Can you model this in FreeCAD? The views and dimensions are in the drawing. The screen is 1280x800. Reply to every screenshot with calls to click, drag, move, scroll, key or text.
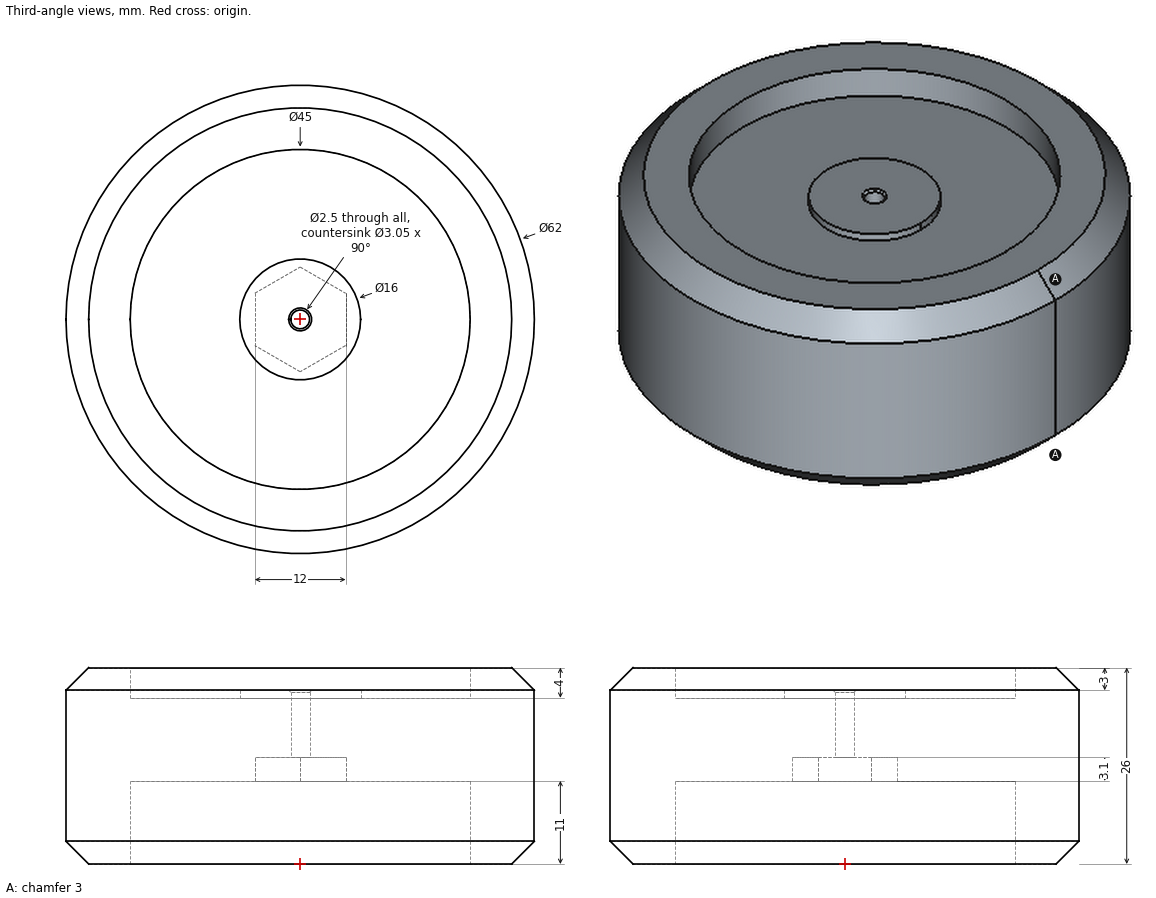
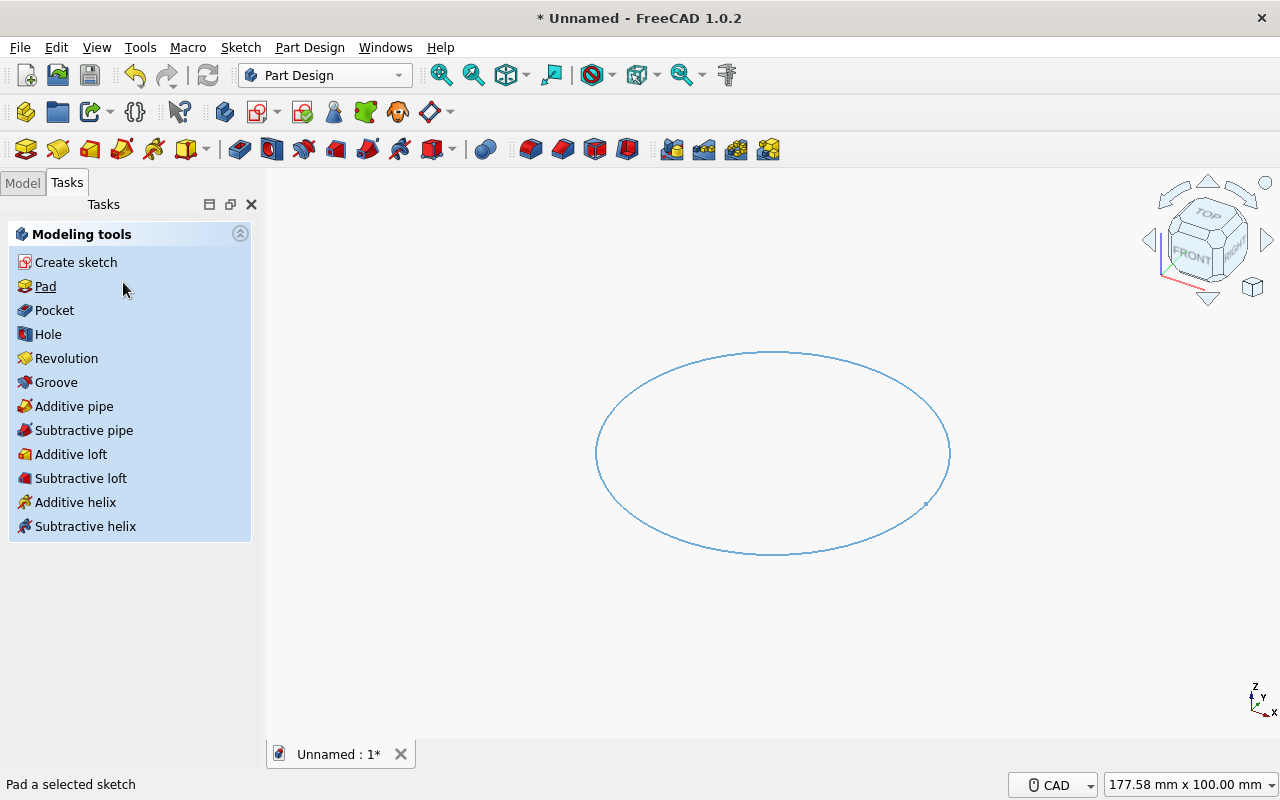
click(26, 150)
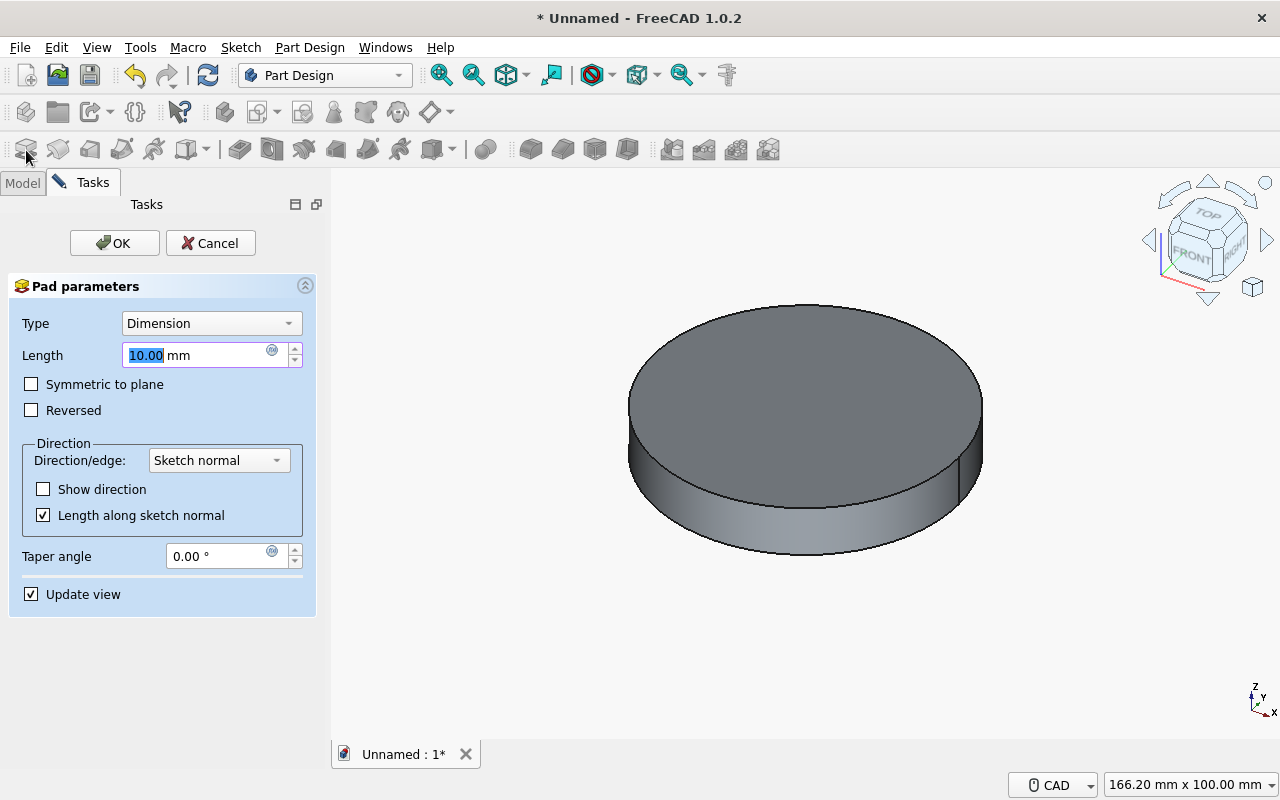
text(26)
key(Tab)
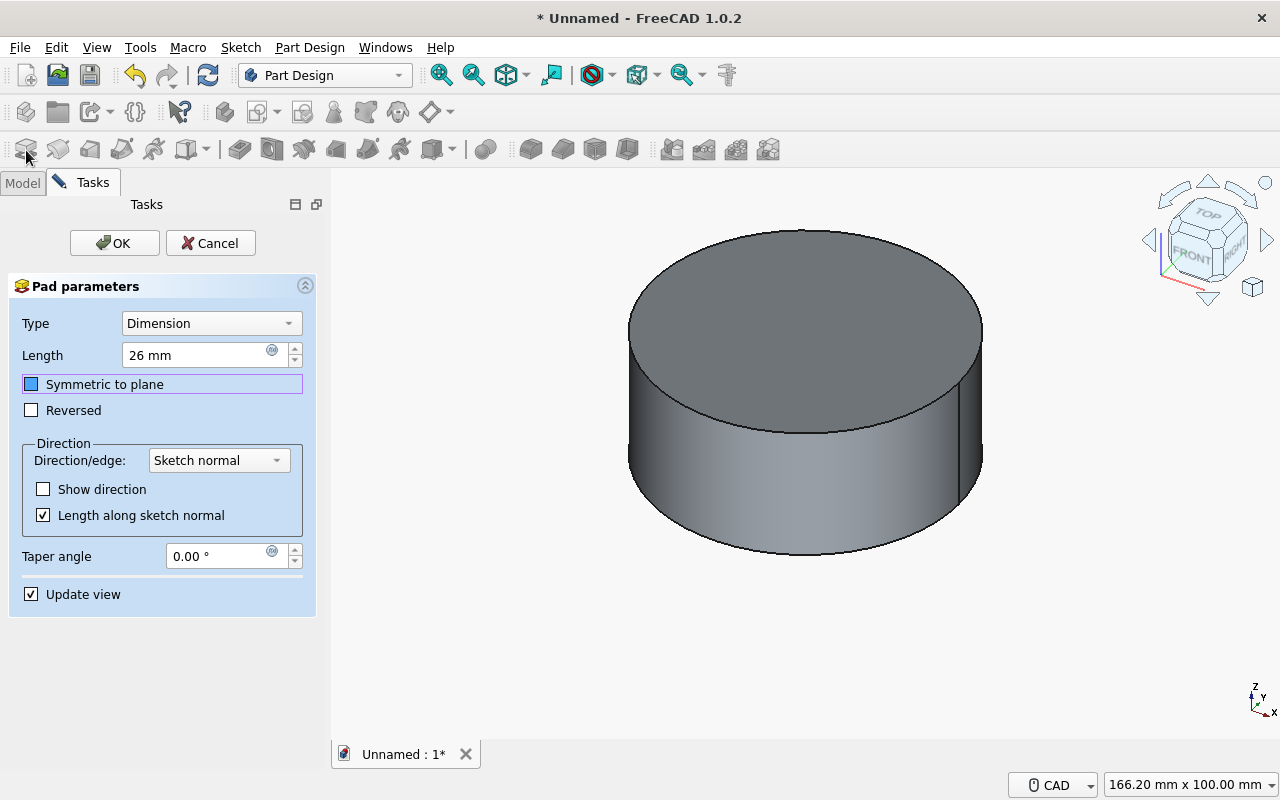
click(115, 243)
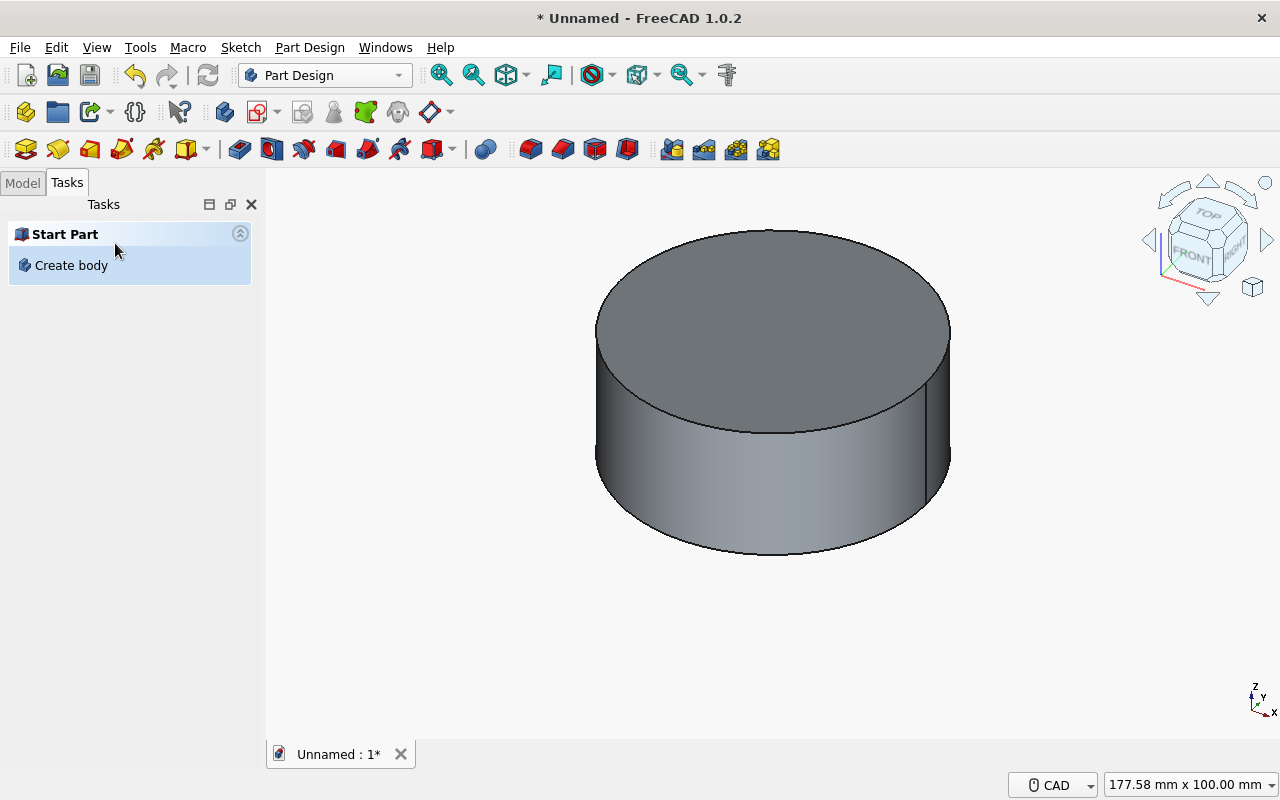
key(5)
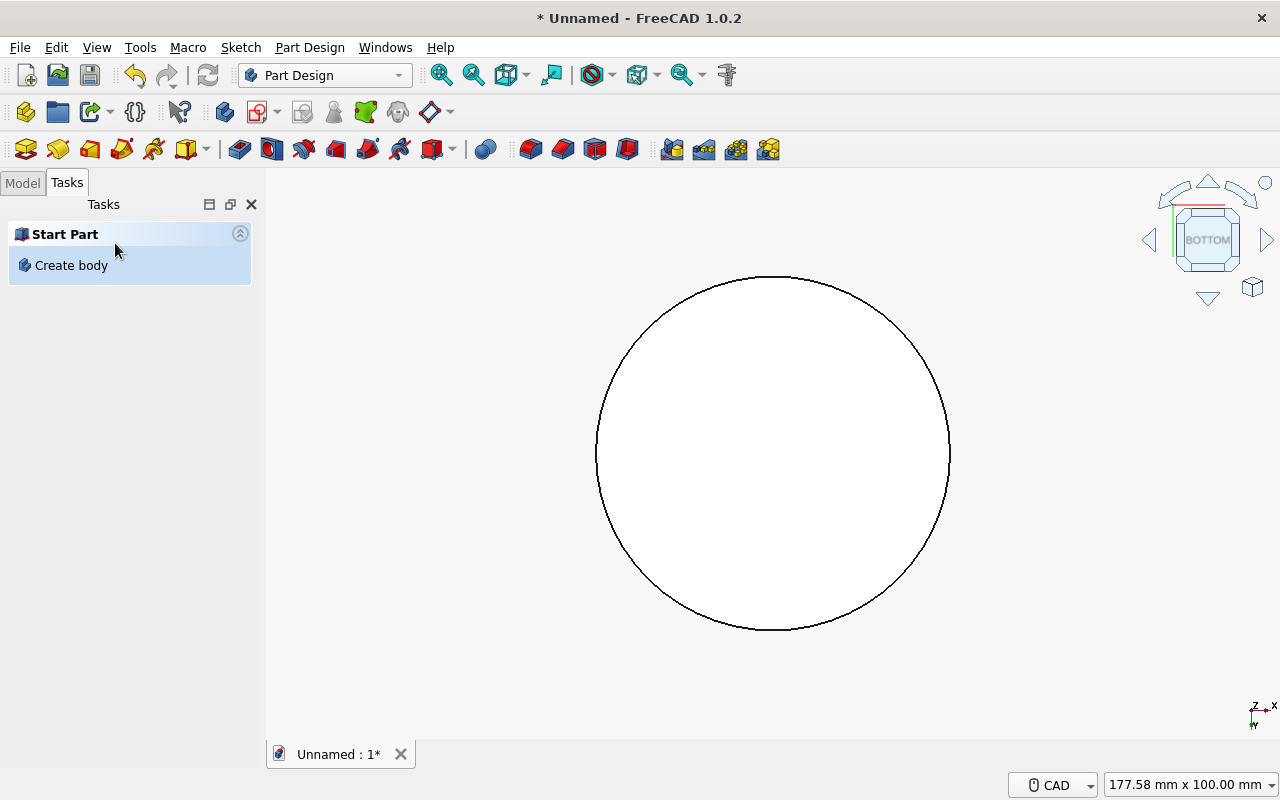
click(773, 452)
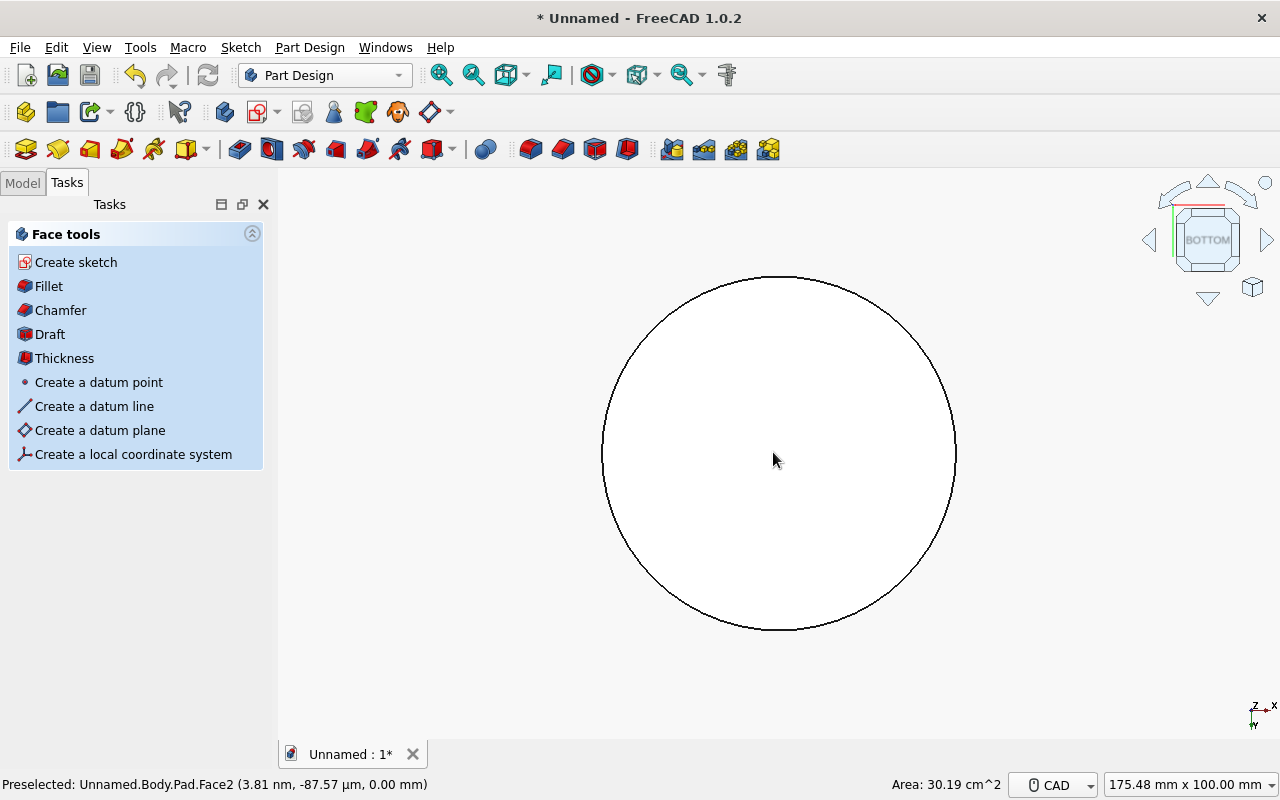
click(258, 112)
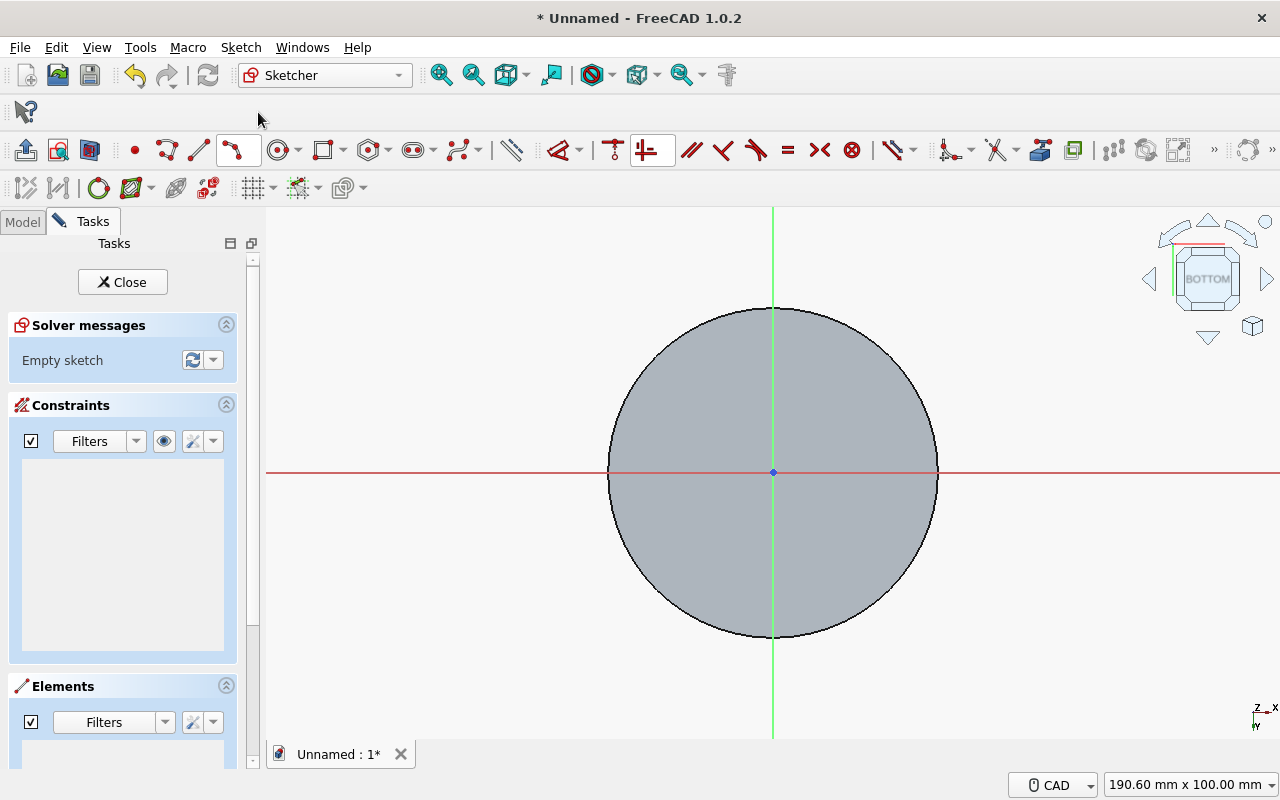
scroll(912, 473, up, 2)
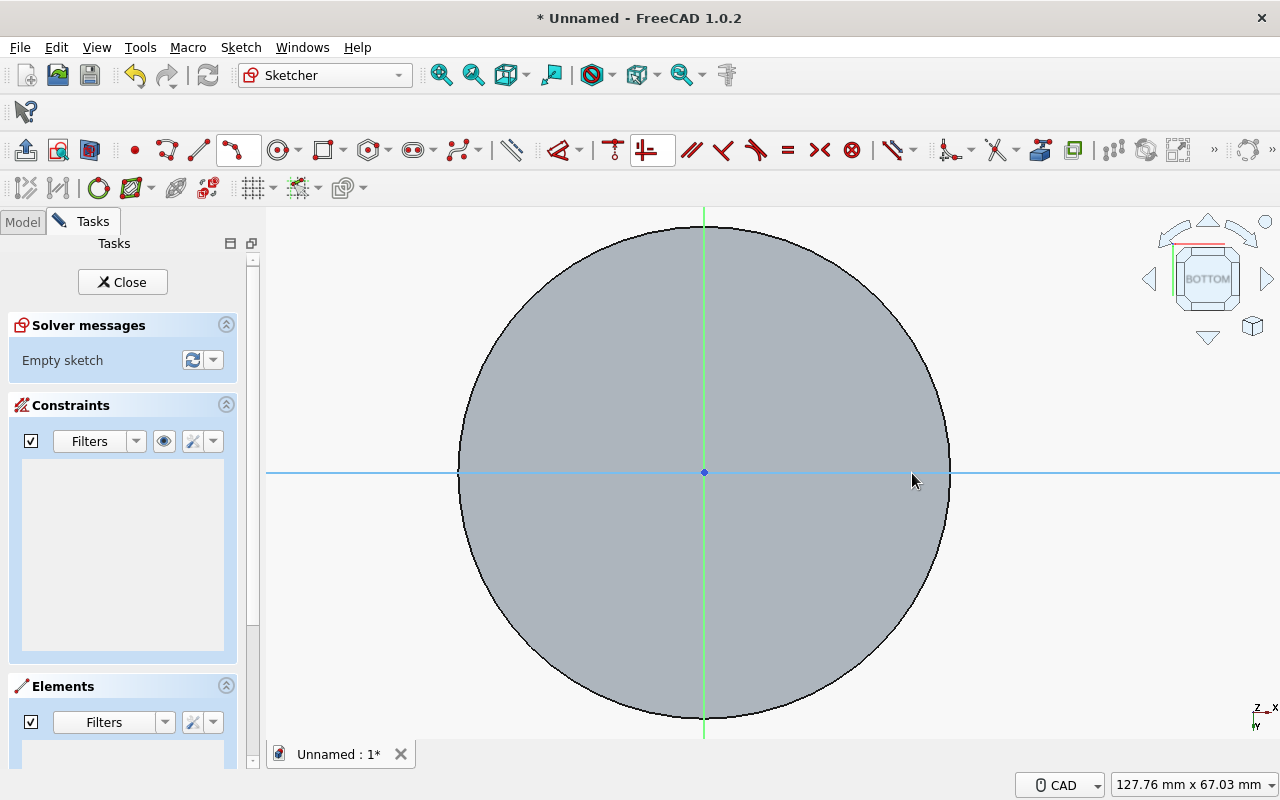
click(278, 150)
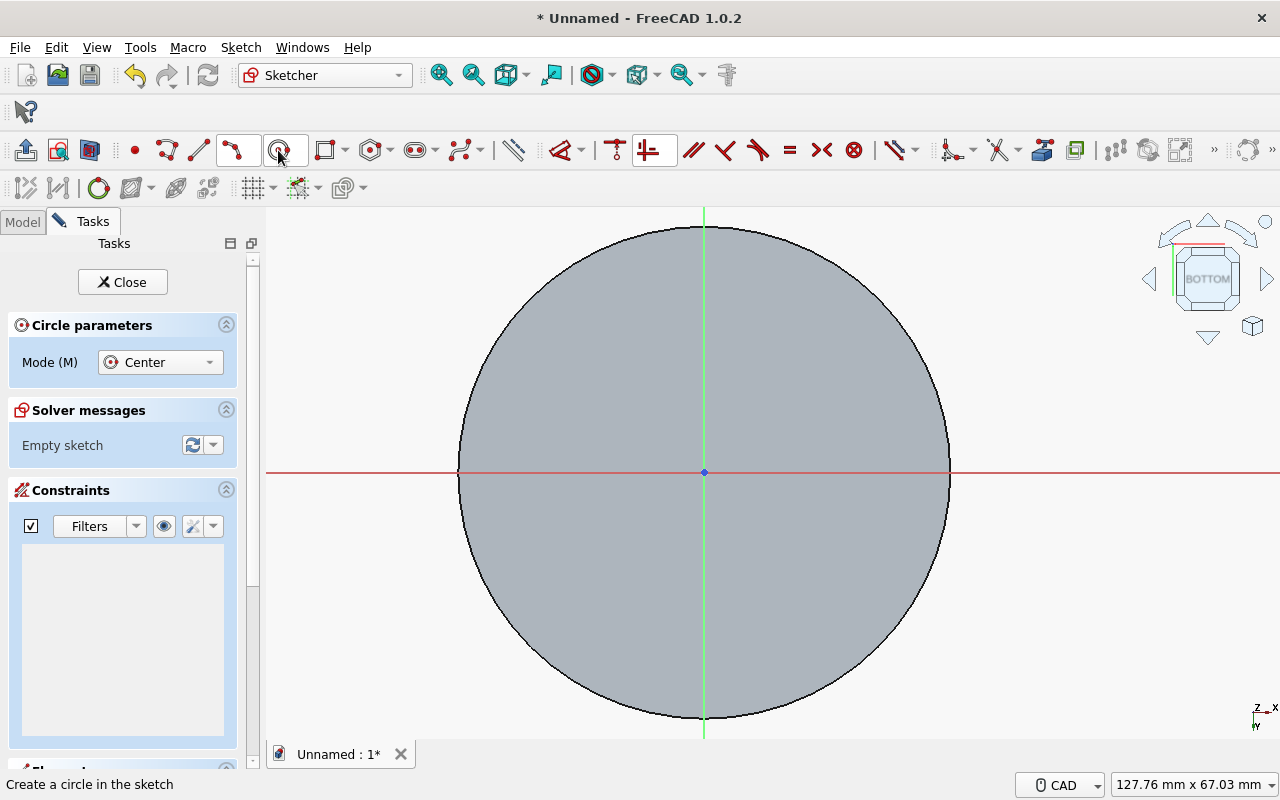
click(704, 473)
click(831, 346)
key(Escape)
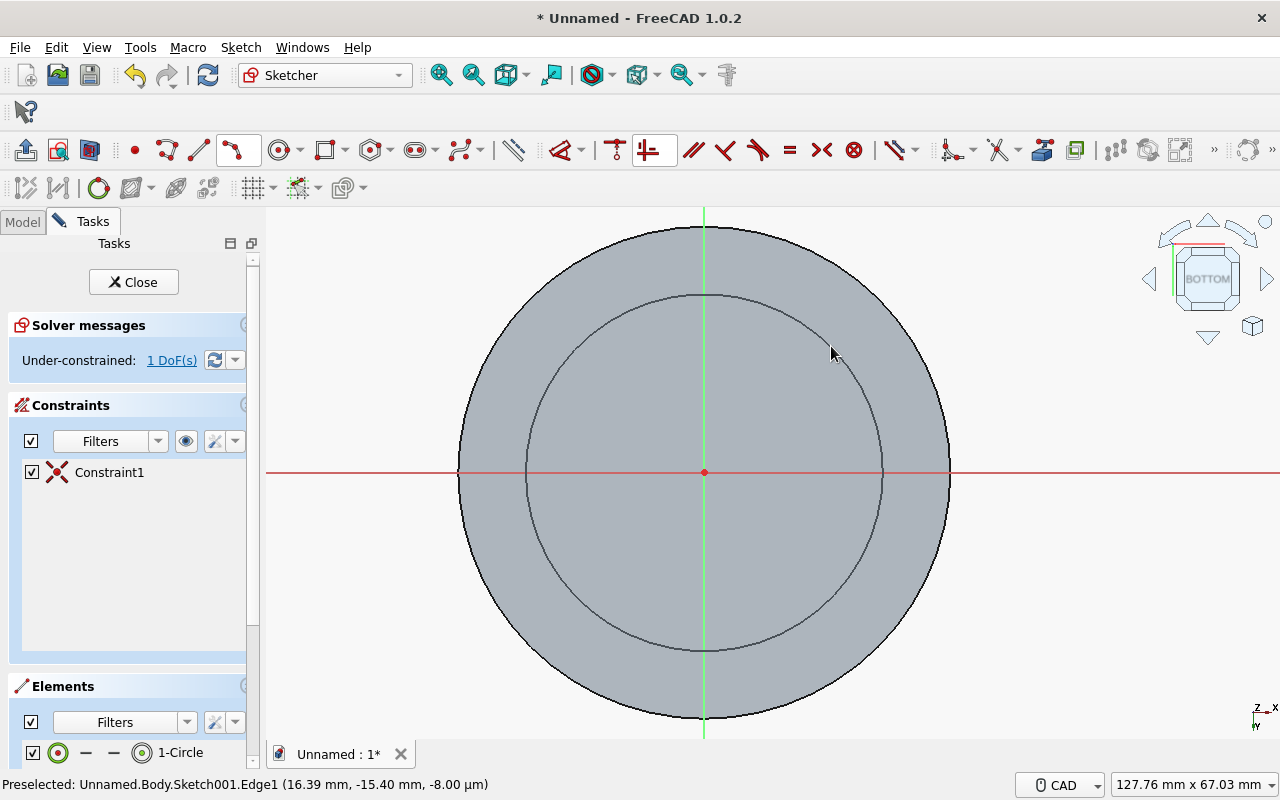
key(d)